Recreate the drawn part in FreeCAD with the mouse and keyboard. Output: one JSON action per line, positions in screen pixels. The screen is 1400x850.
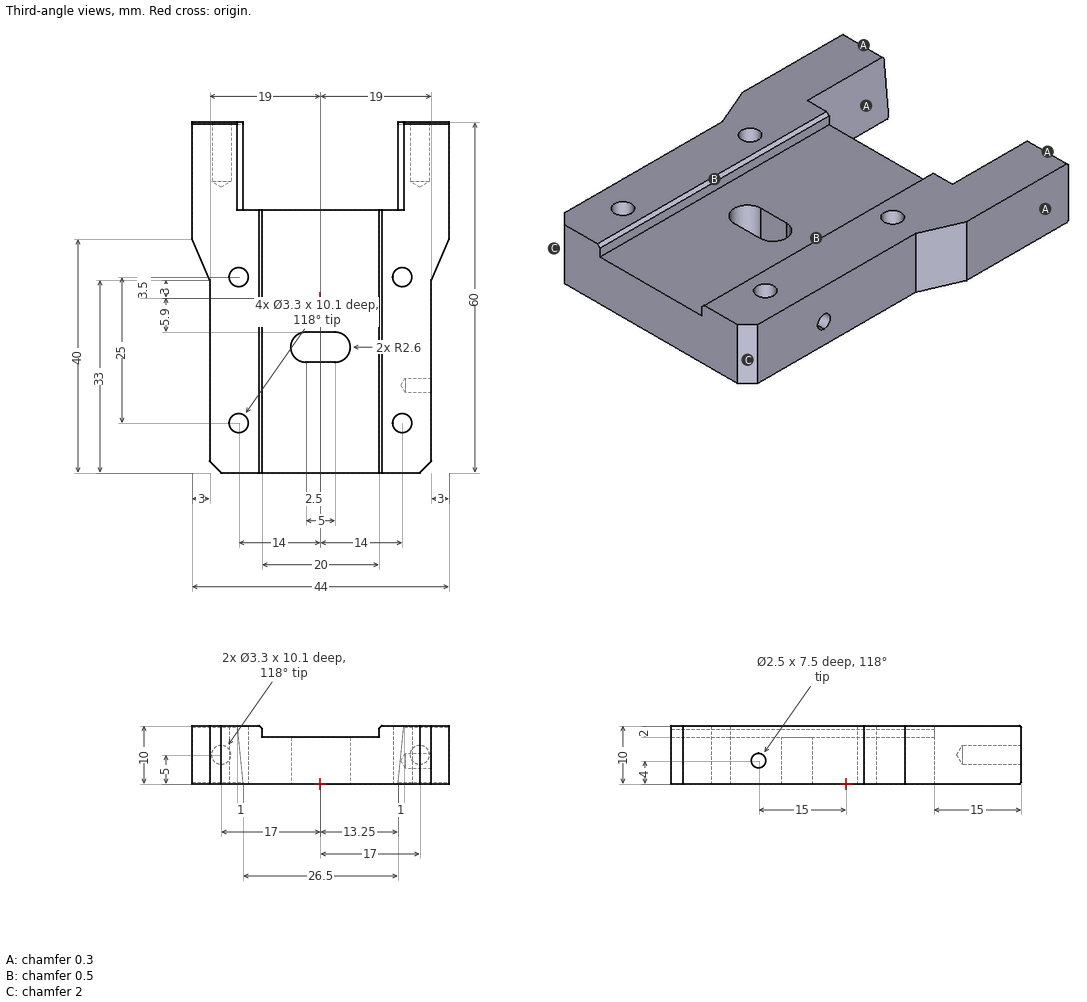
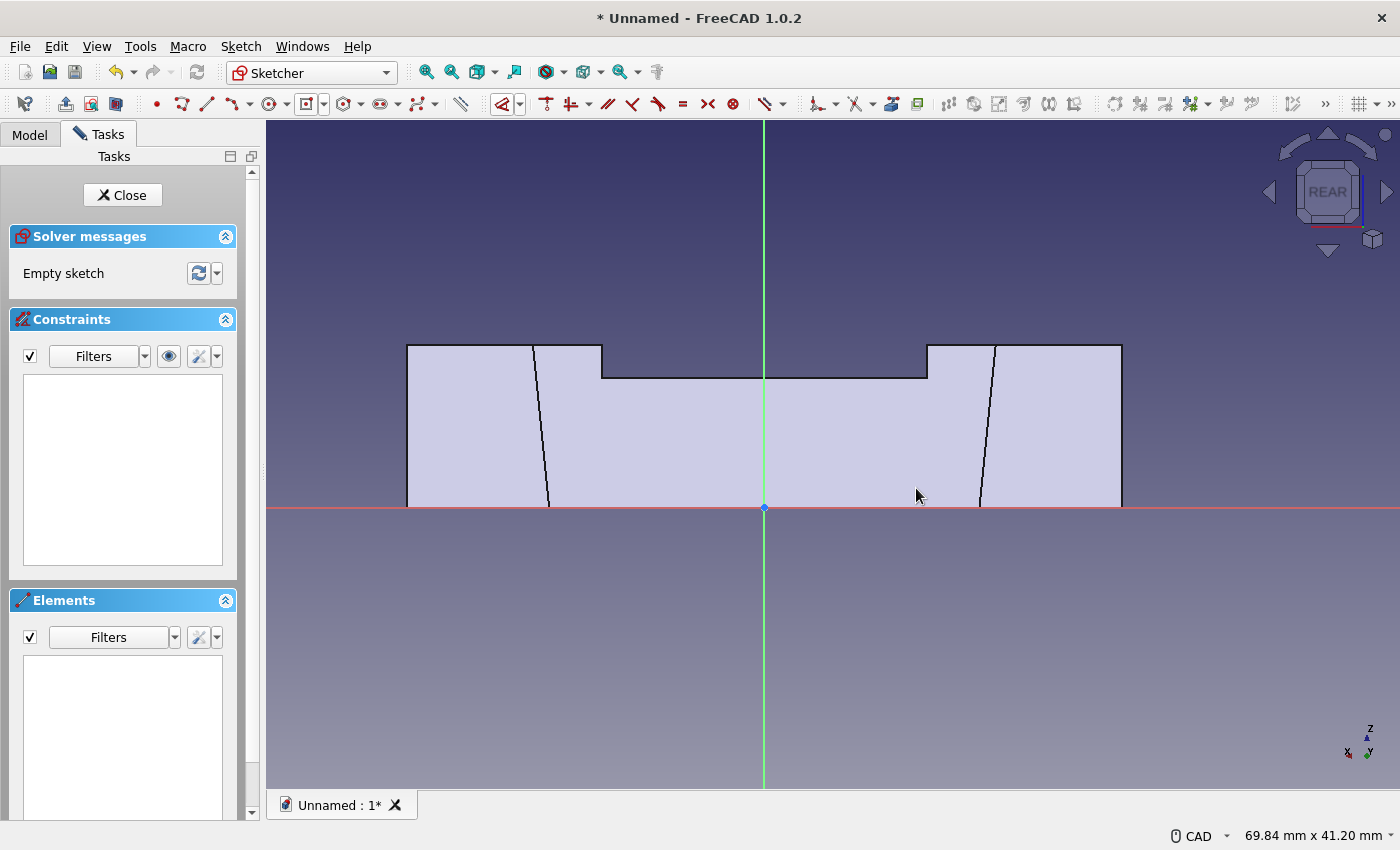
{"action": "left_click", "coordinate": [268, 104]}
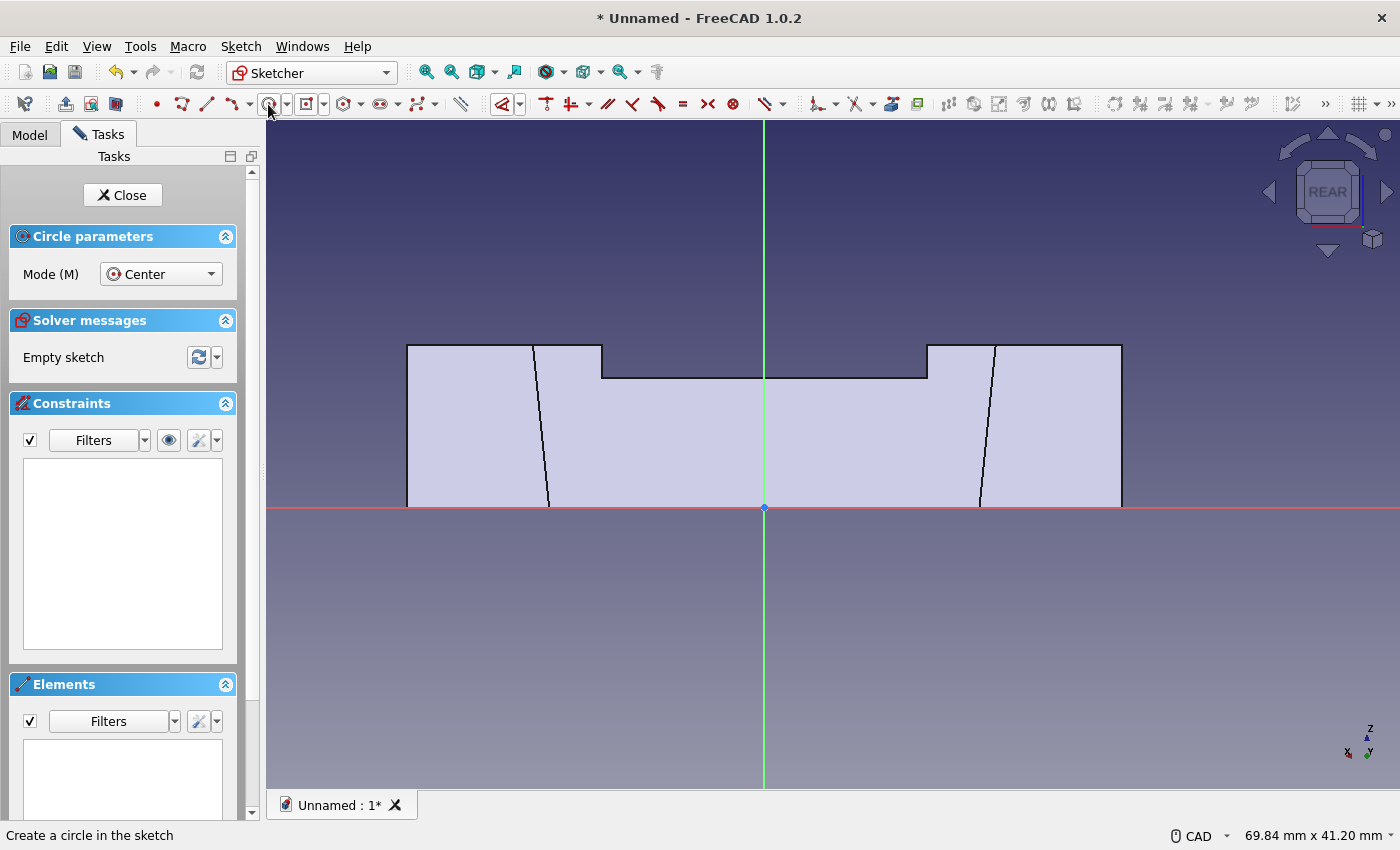
{"action": "left_click", "coordinate": [1040, 427]}
{"action": "left_click", "coordinate": [1059, 408]}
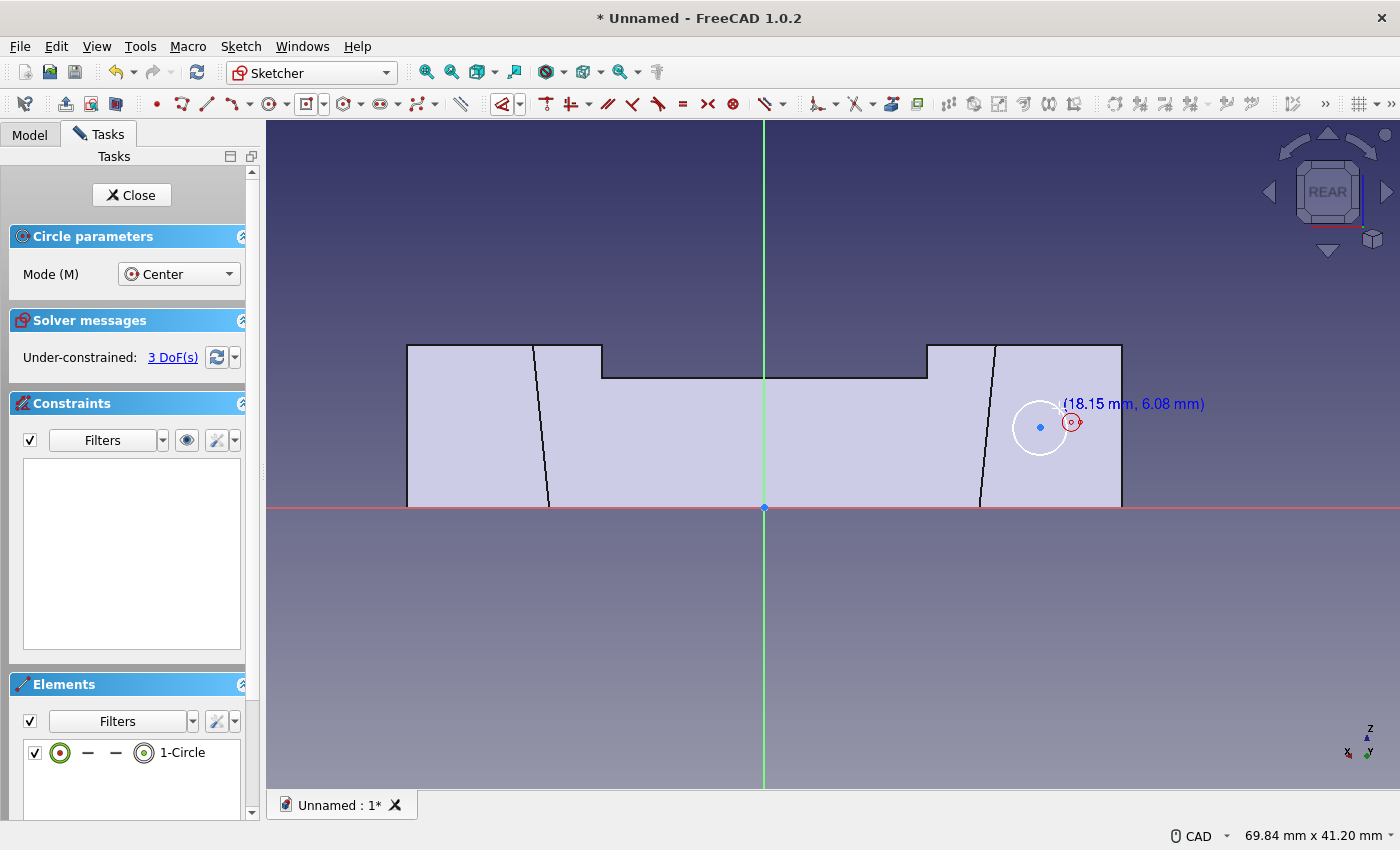
{"action": "left_click", "coordinate": [488, 427]}
{"action": "left_click", "coordinate": [507, 408]}
{"action": "key", "text": "Escape"}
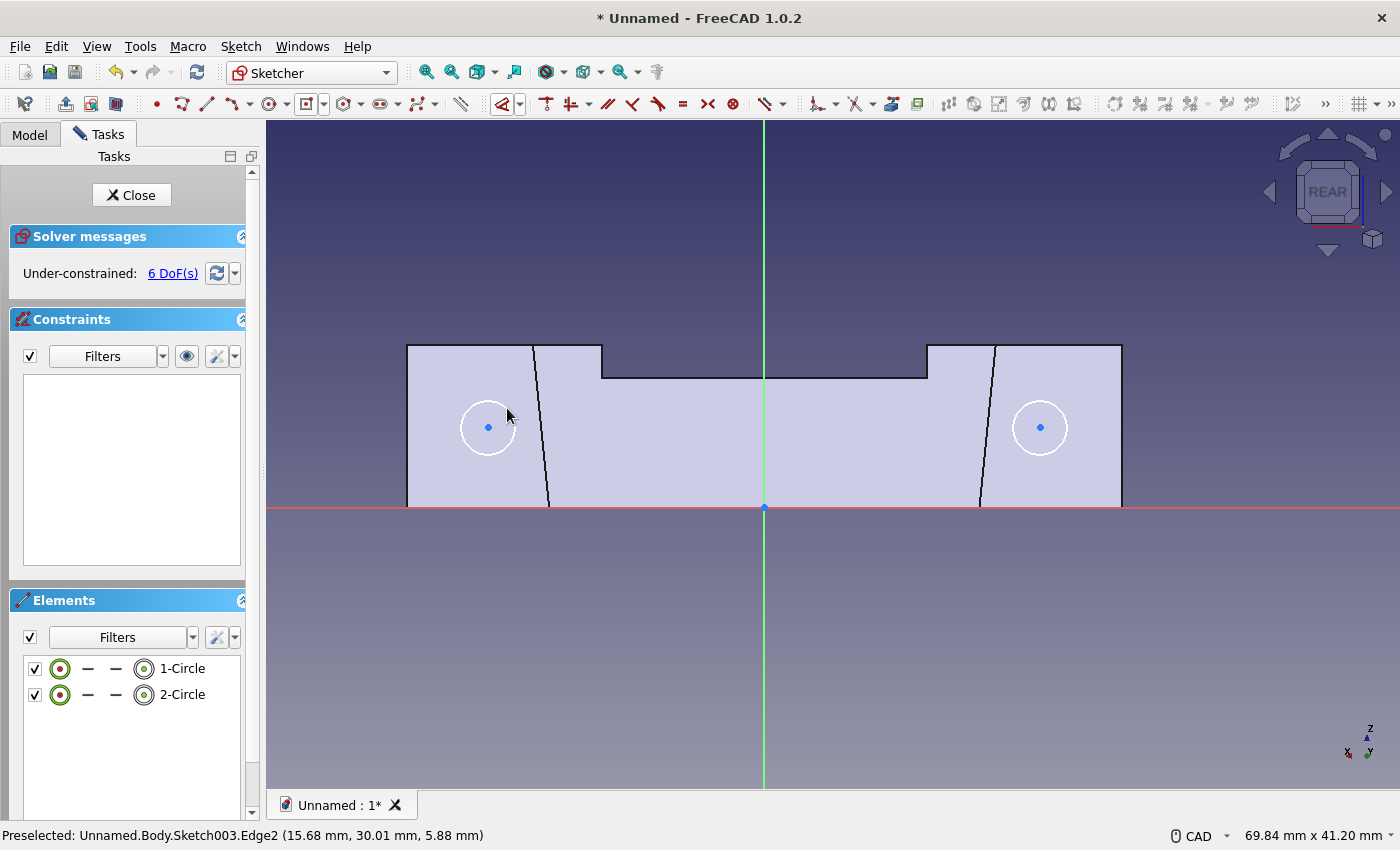
{"action": "left_click", "coordinate": [1059, 409]}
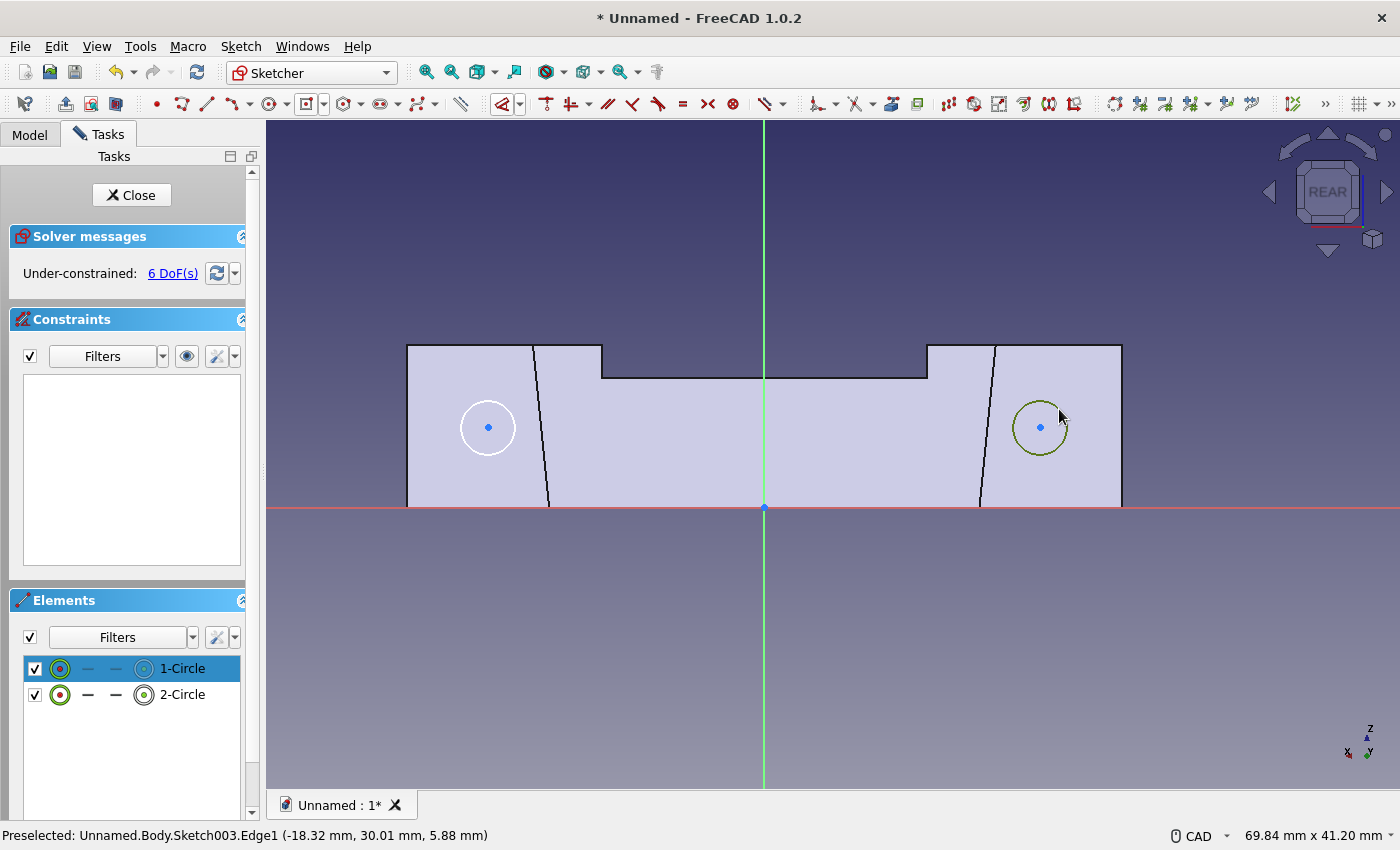
{"action": "left_click", "coordinate": [507, 409]}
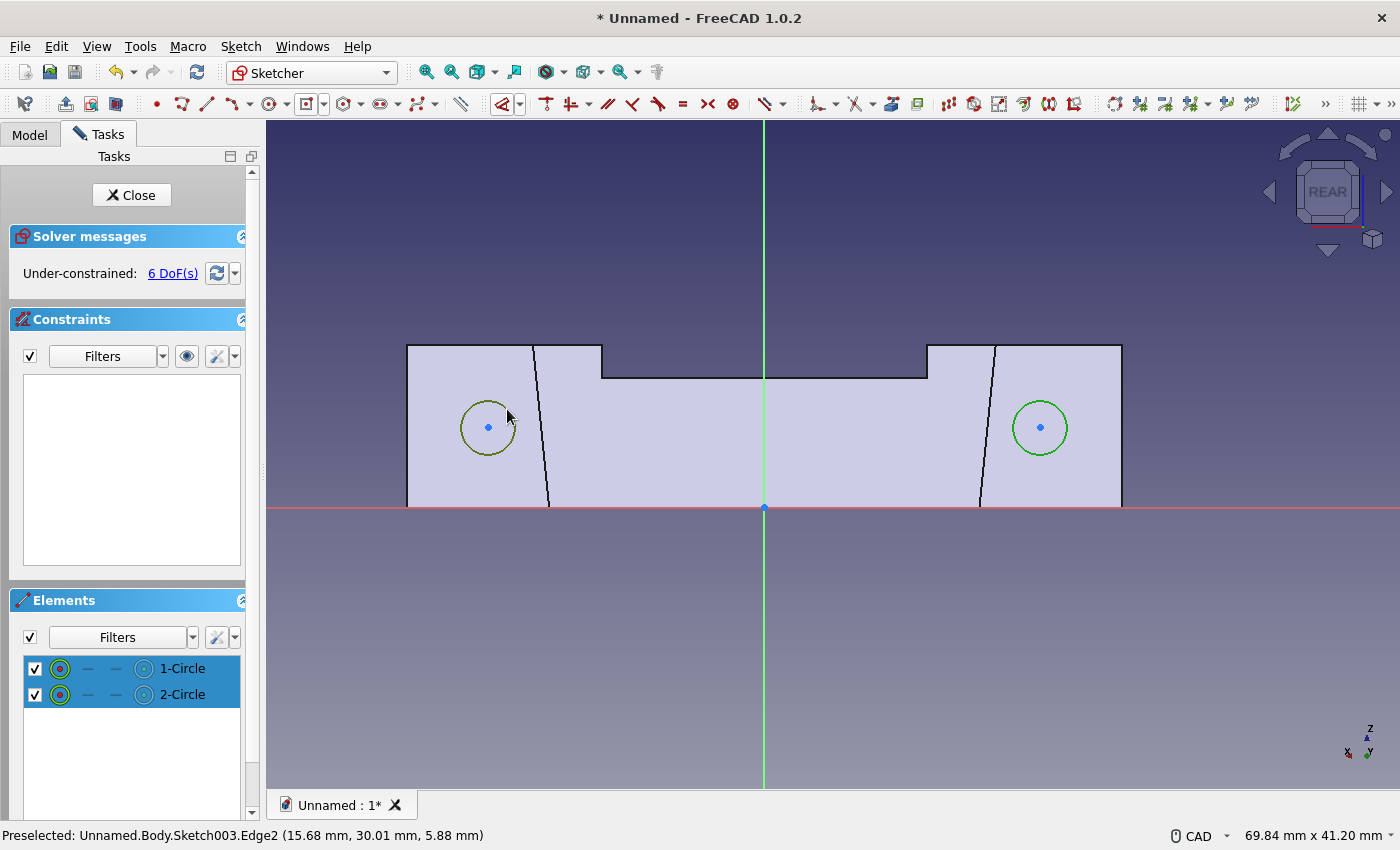
{"action": "left_click", "coordinate": [683, 104]}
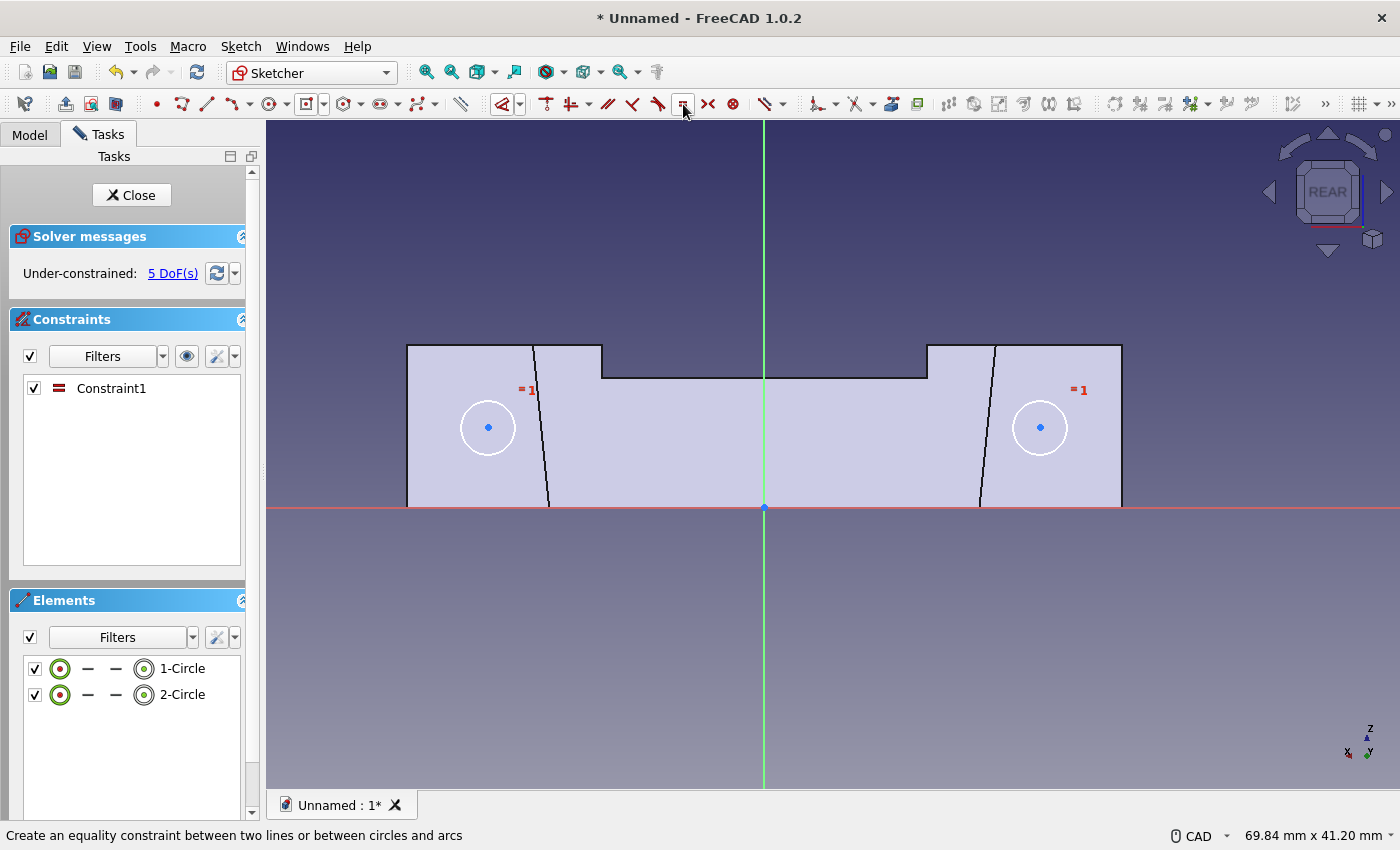
{"action": "left_click", "coordinate": [1059, 409]}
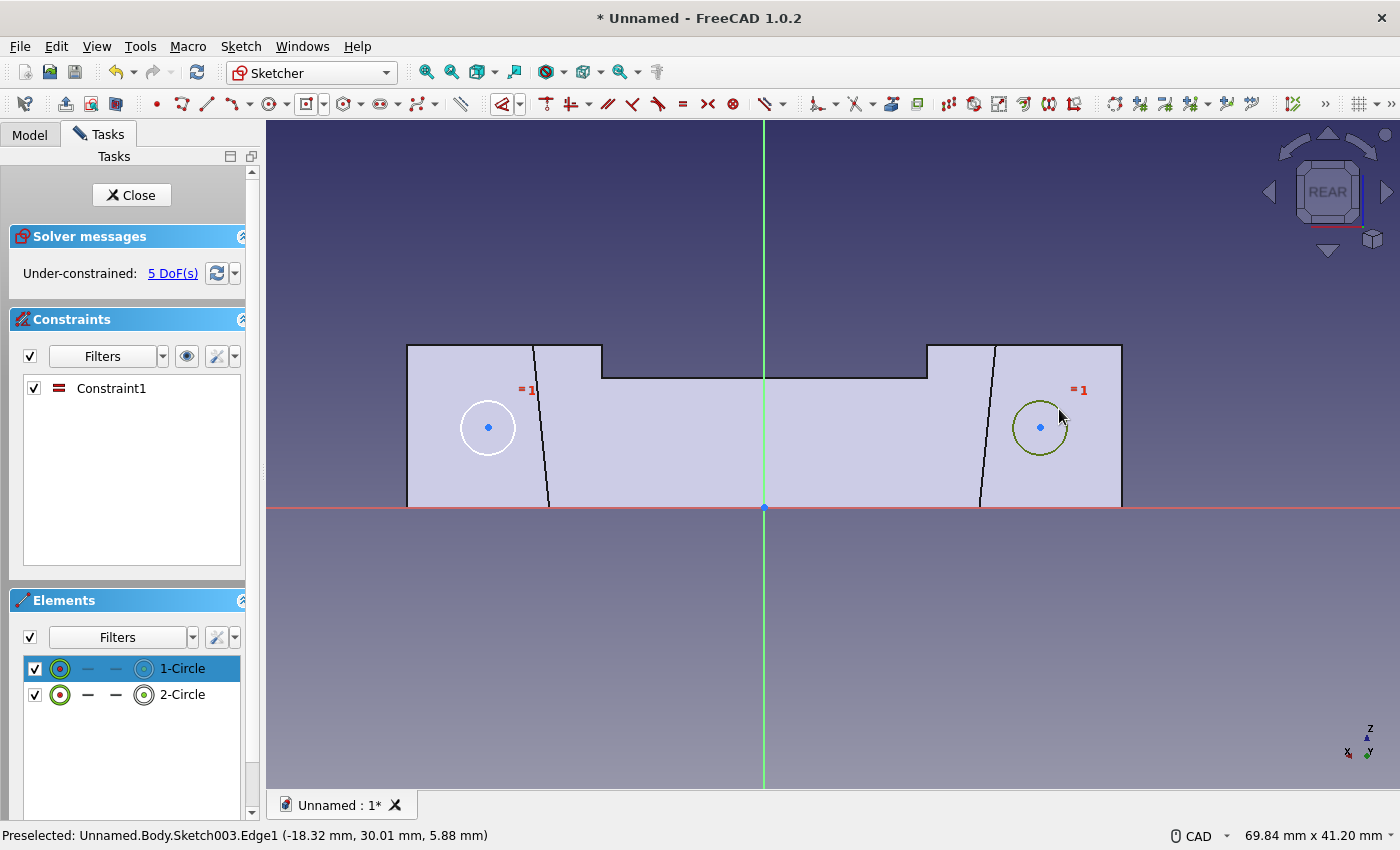
{"action": "left_click", "coordinate": [520, 104]}